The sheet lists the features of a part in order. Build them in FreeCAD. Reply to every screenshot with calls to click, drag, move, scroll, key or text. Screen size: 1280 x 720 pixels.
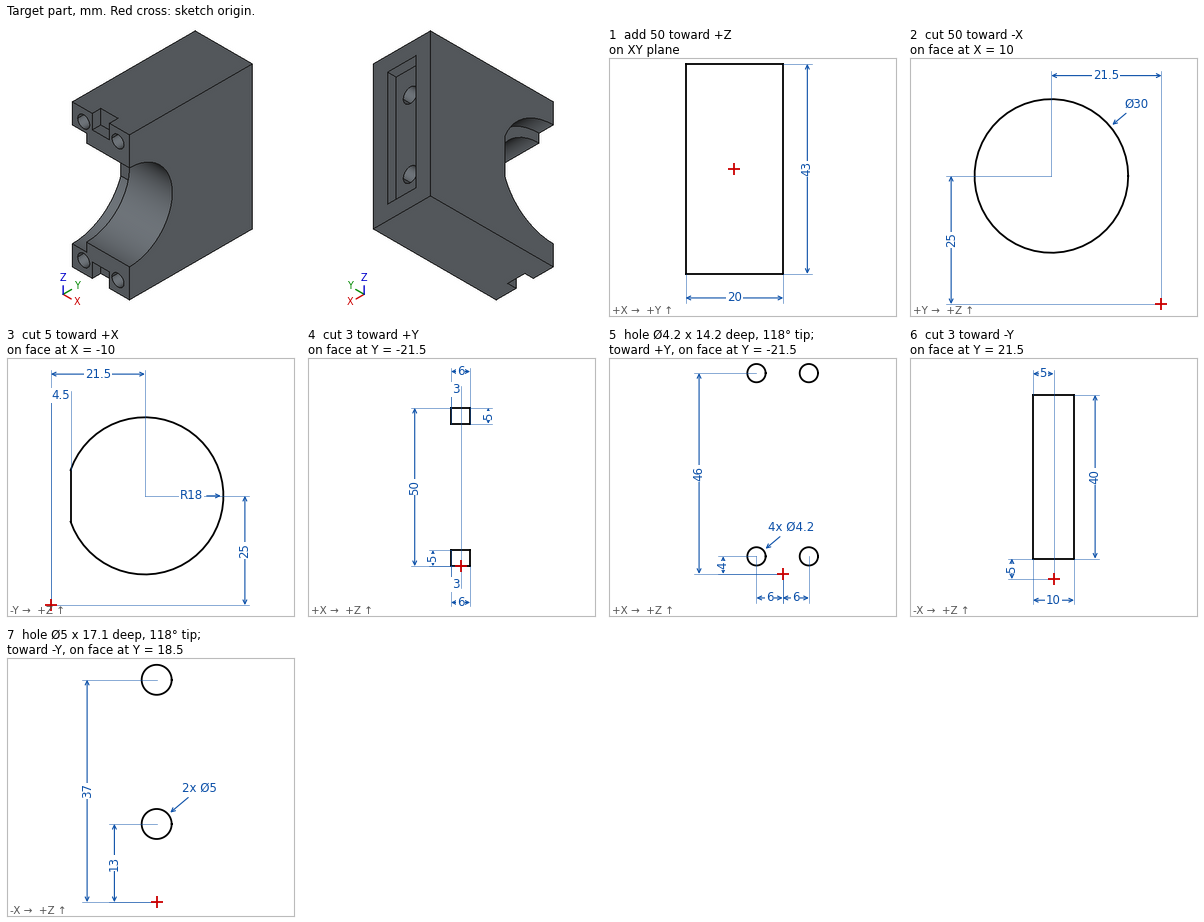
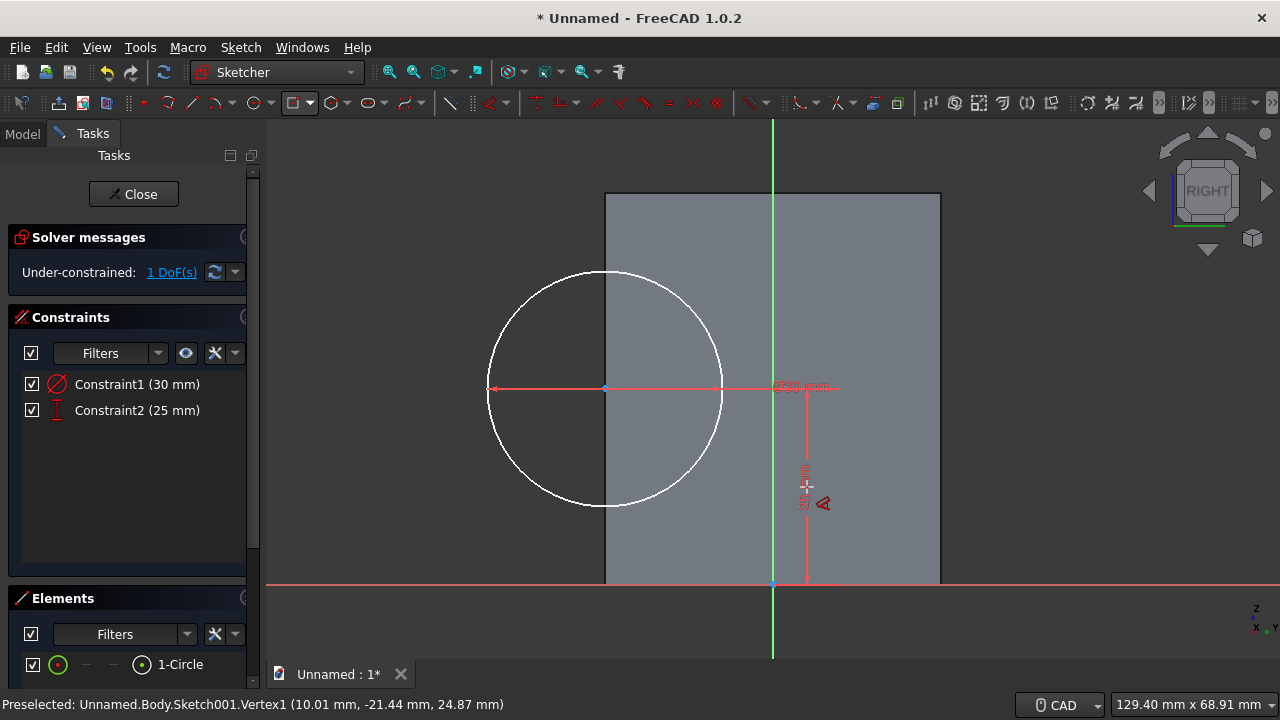
click(605, 389)
click(689, 619)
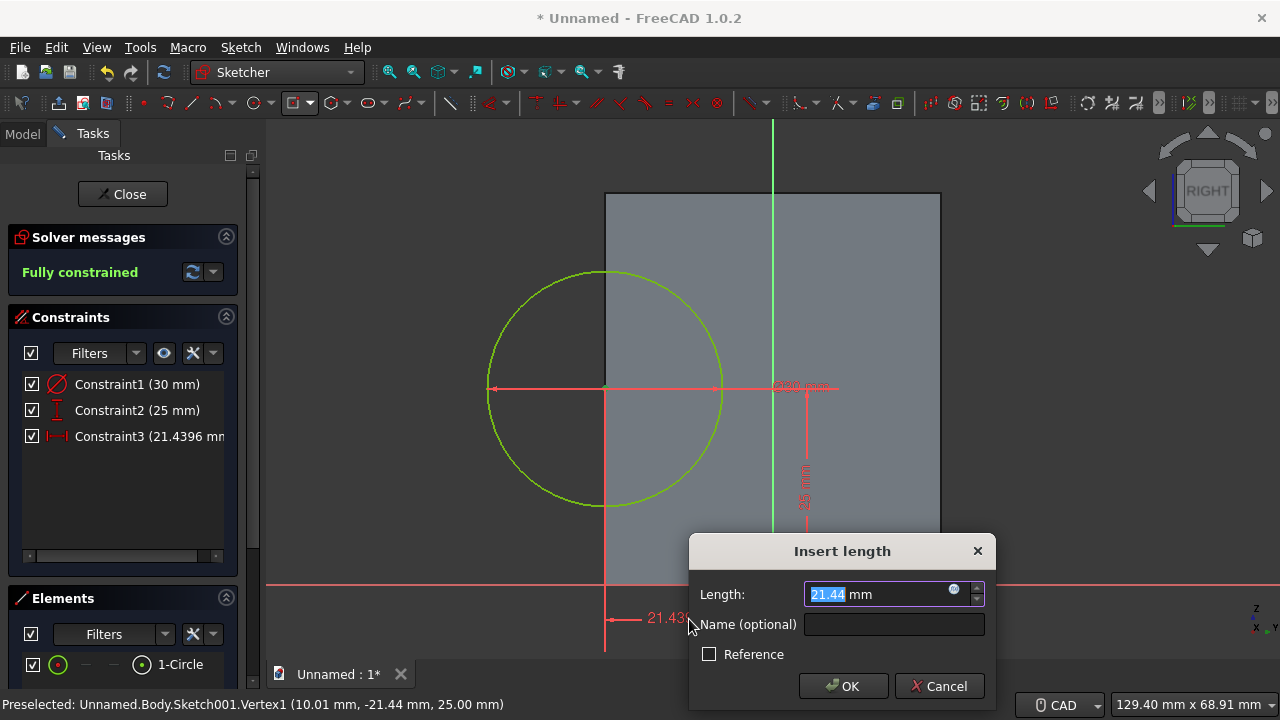
text(21.5)
key(Return)
key(Escape)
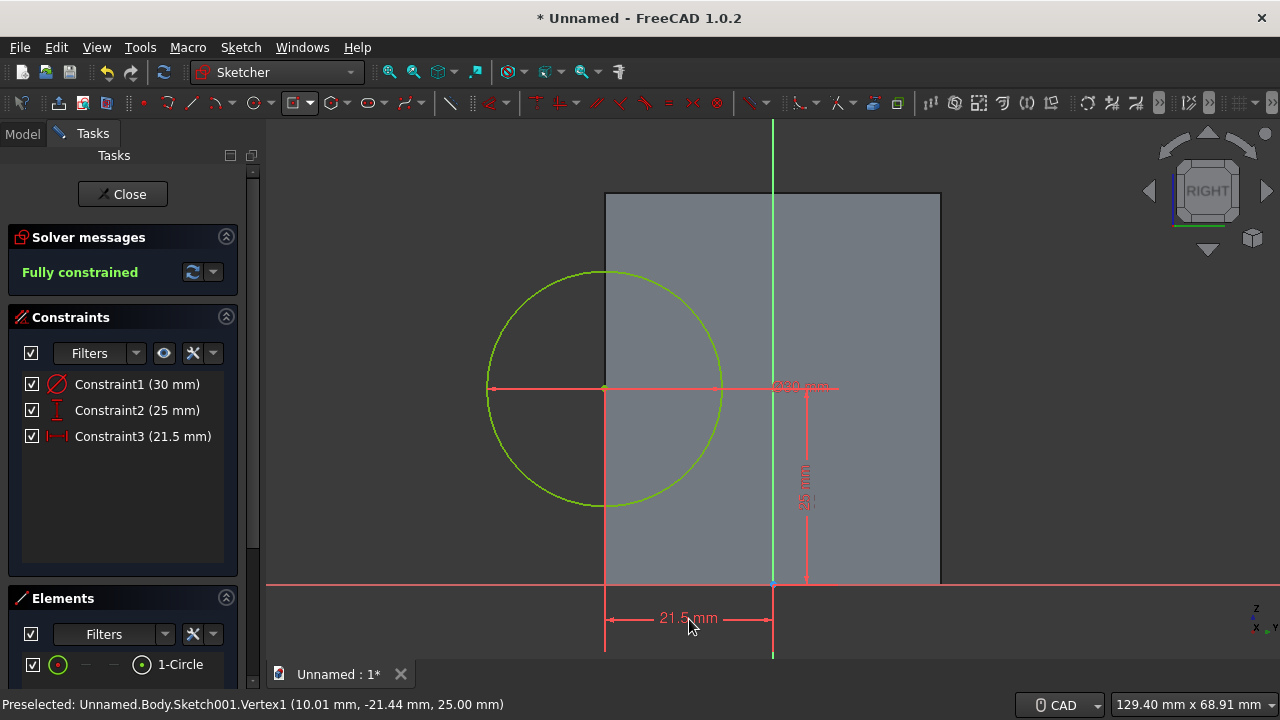
click(123, 194)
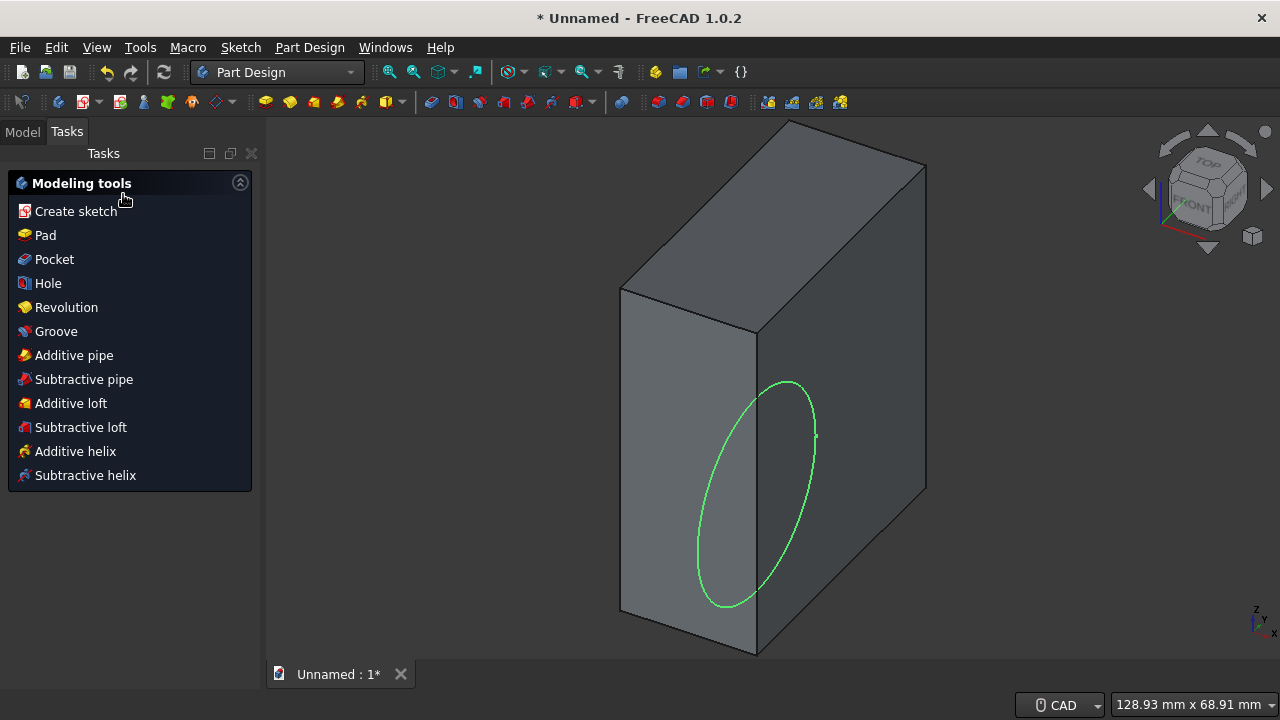
click(432, 102)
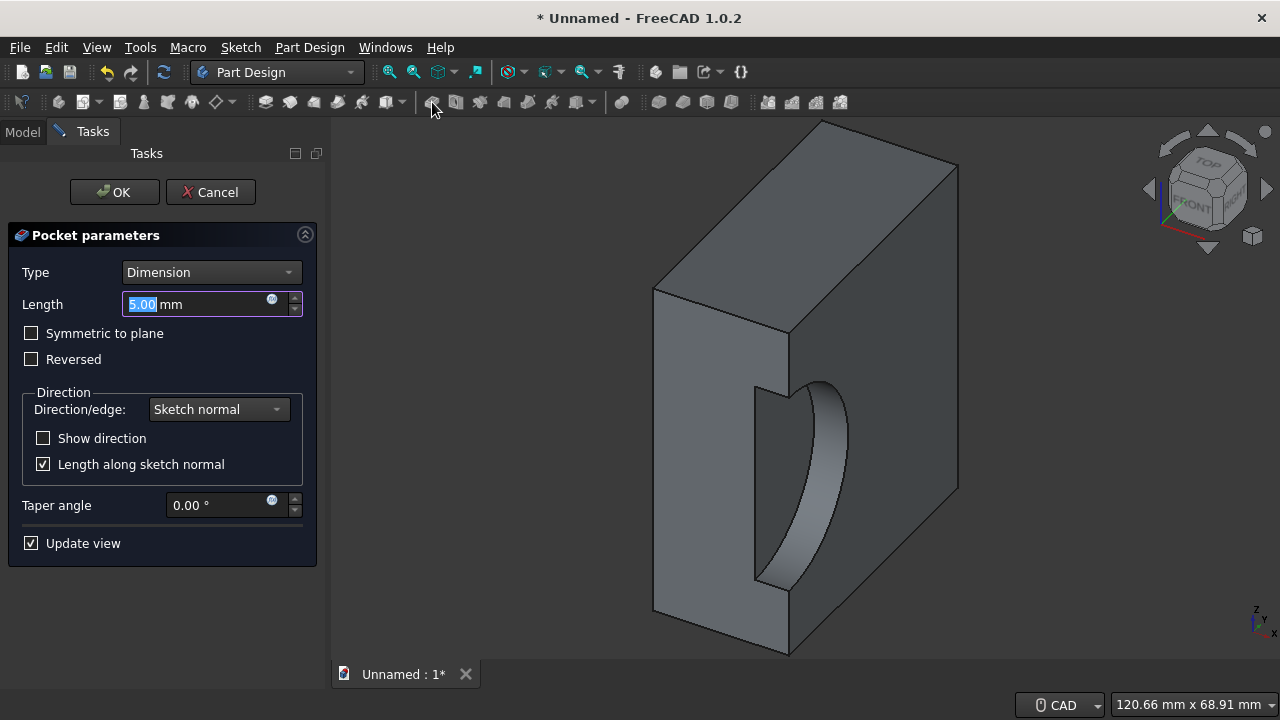
text(50)
key(Tab)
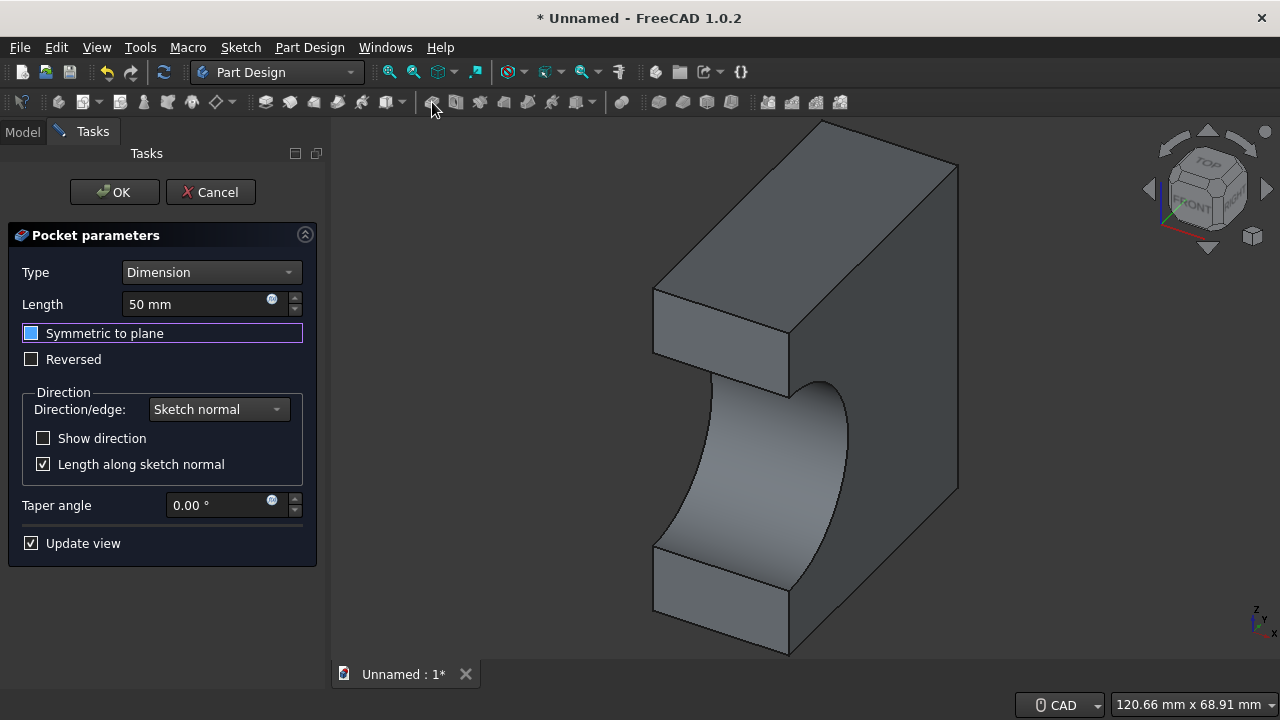
click(115, 192)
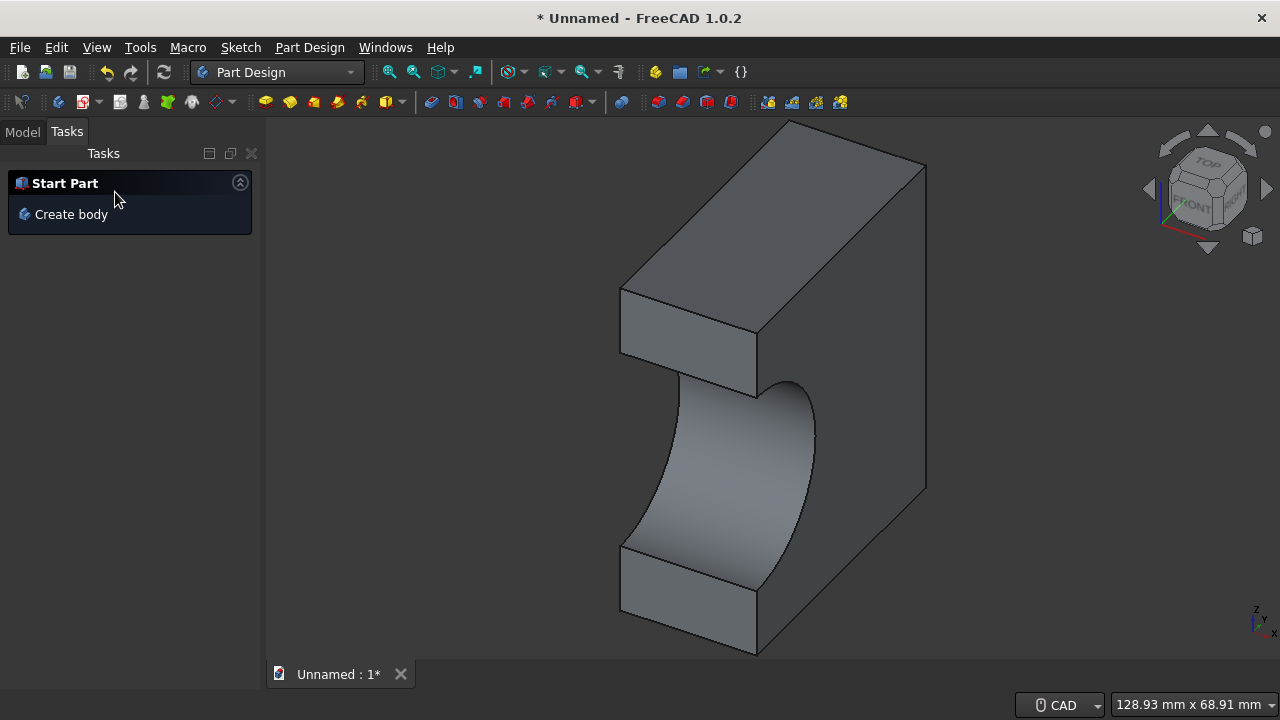
key(6)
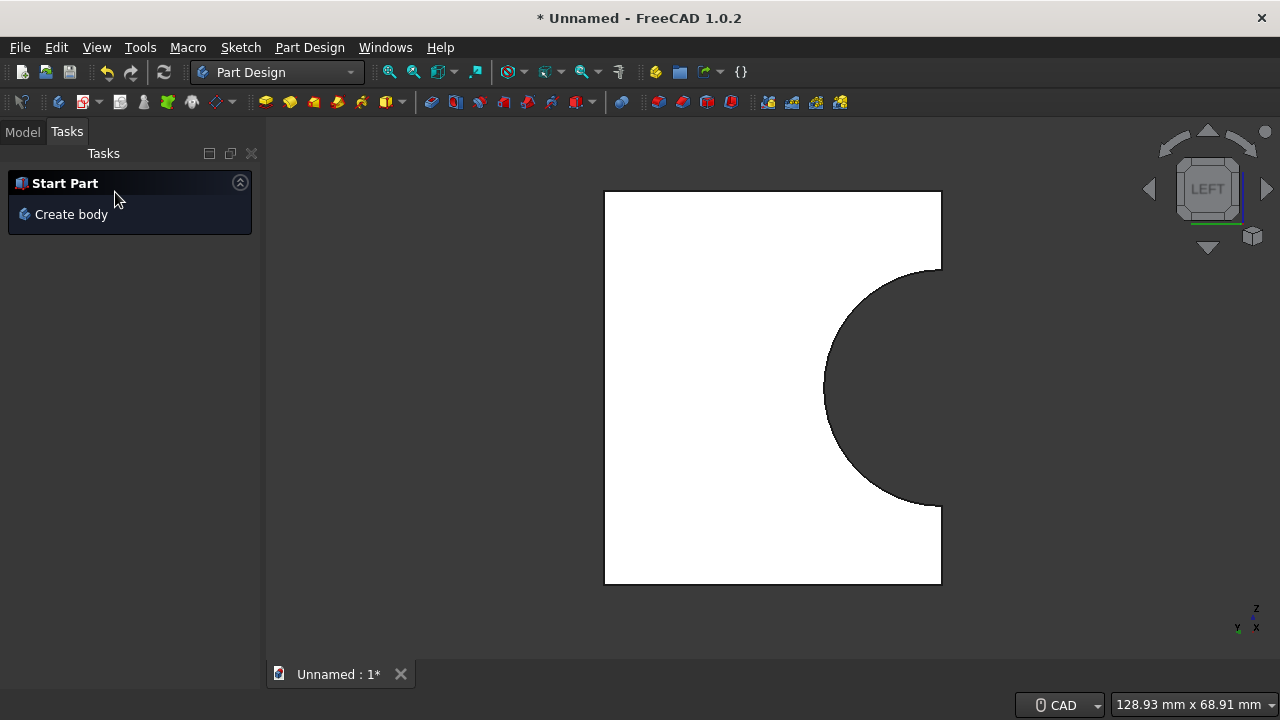
click(725, 443)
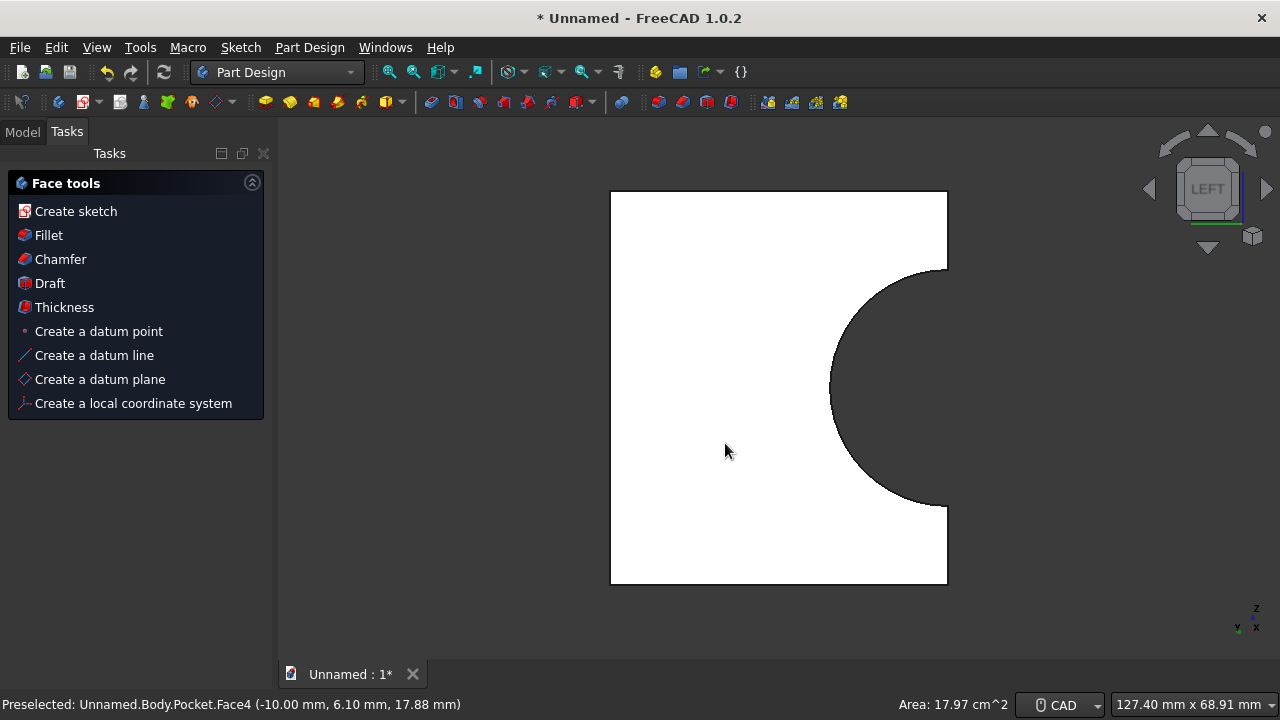
click(84, 102)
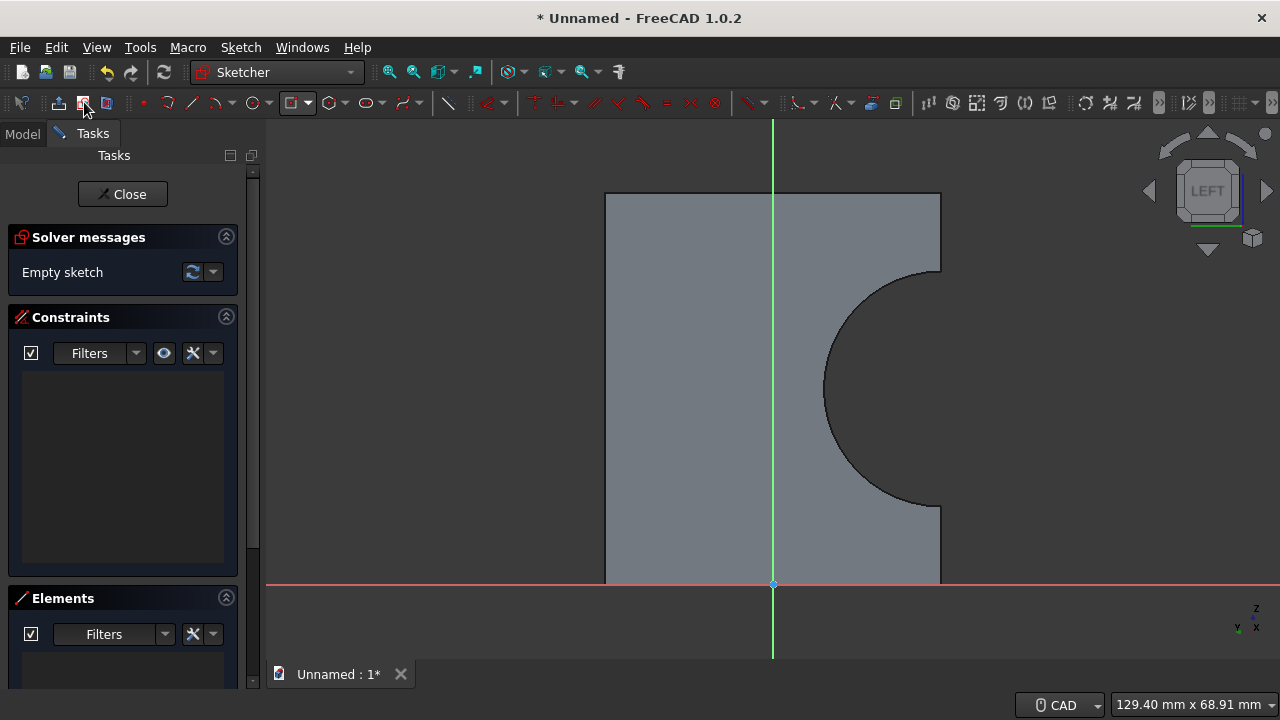
scroll(1115, 616, up, 2)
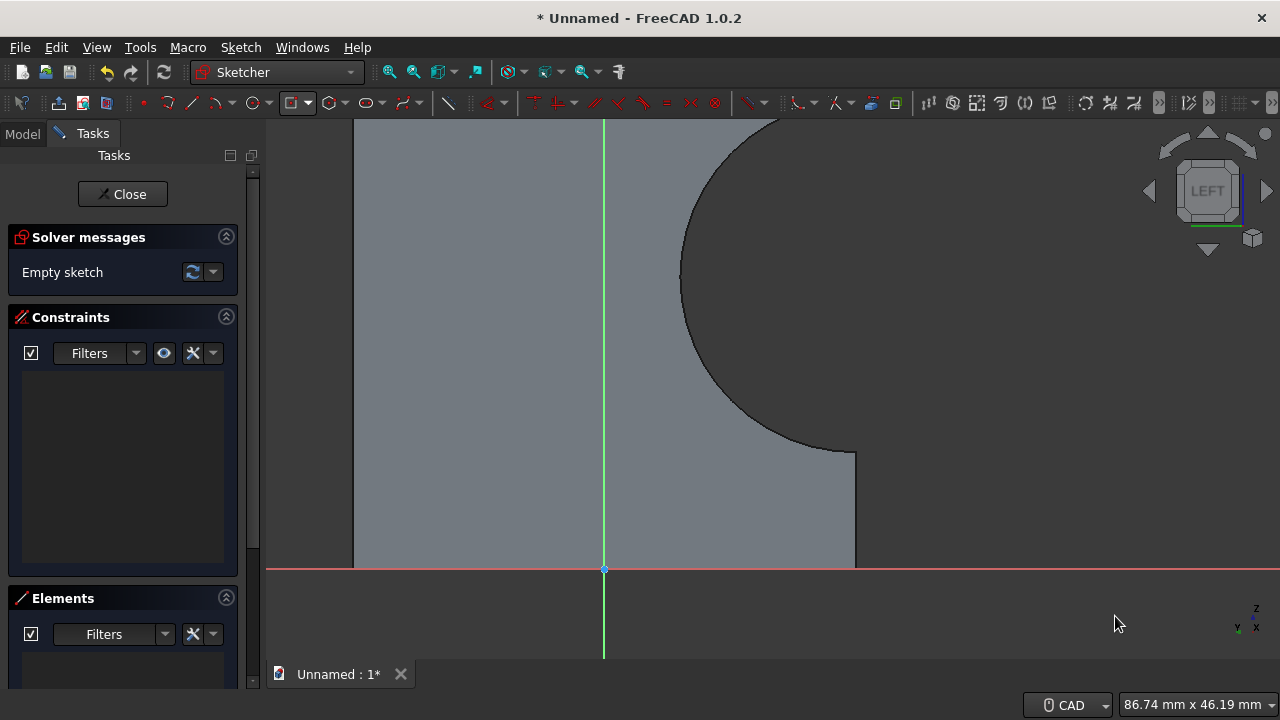
click(192, 104)